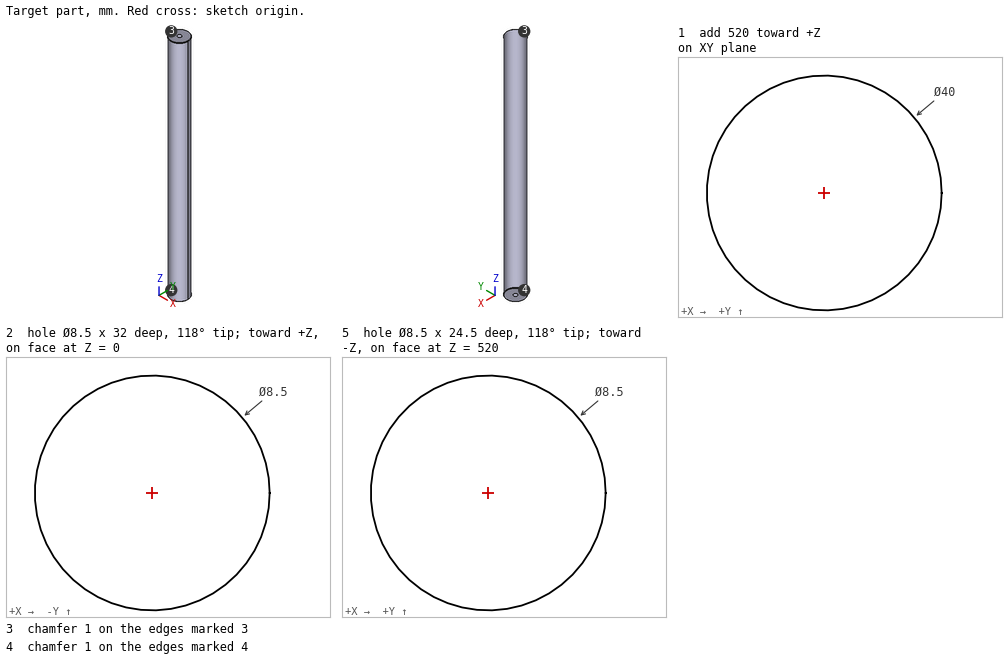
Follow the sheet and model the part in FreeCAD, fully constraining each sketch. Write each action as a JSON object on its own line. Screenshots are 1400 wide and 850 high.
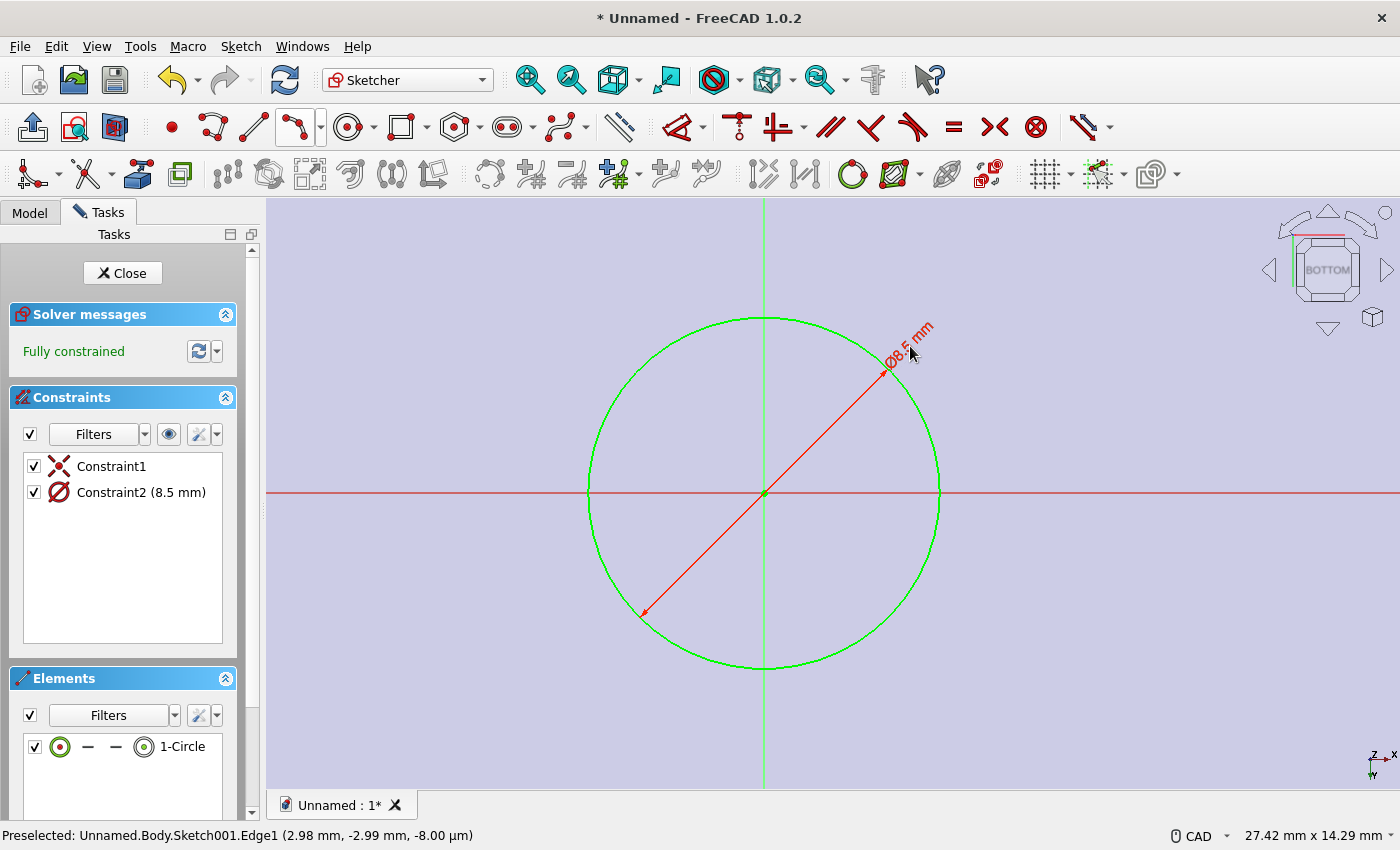
{"action": "left_click", "coordinate": [123, 273]}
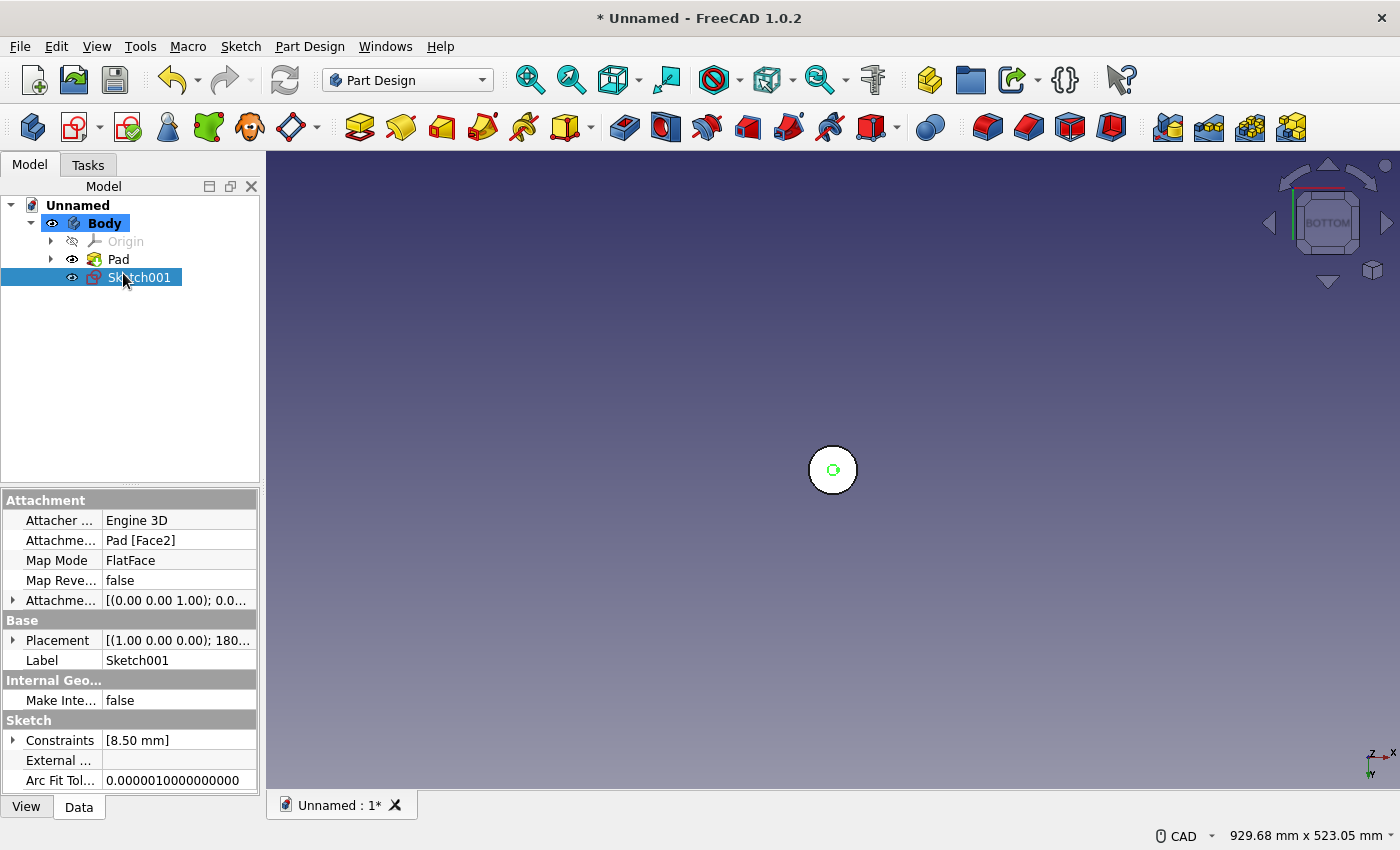
{"action": "left_click", "coordinate": [666, 128]}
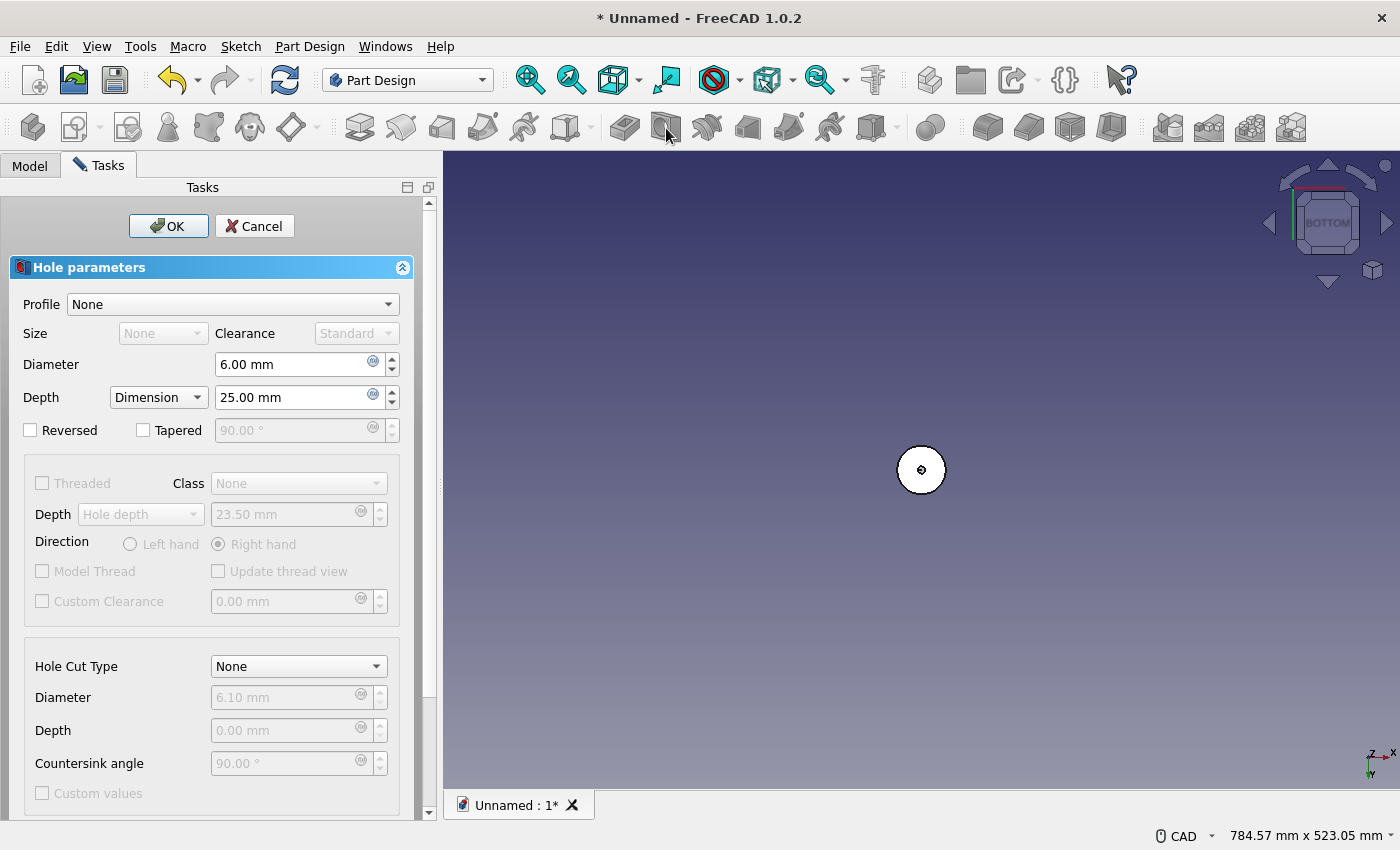
{"action": "triple_click", "coordinate": [300, 364]}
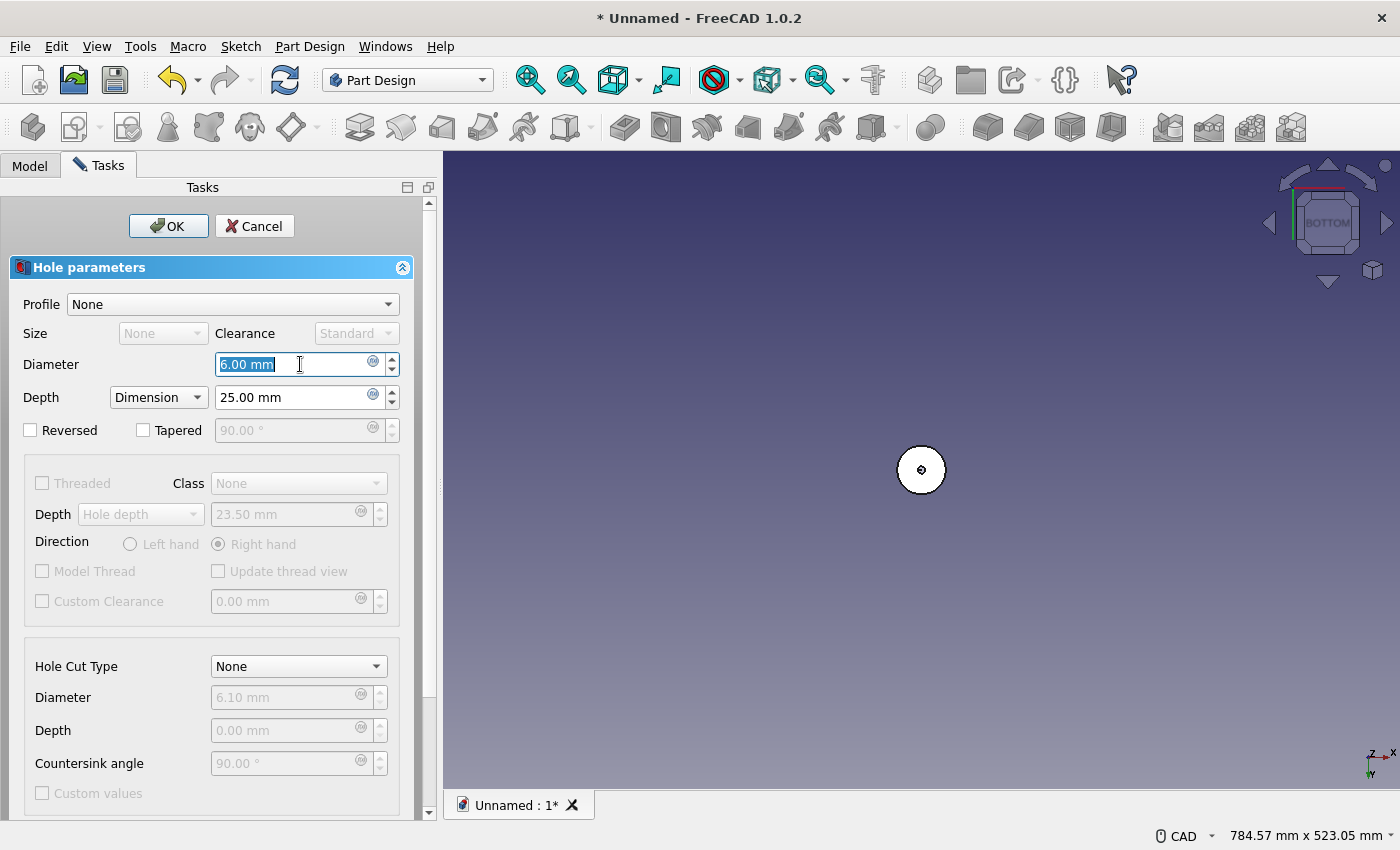
{"action": "type", "text": "8.5"}
{"action": "key", "text": "Tab"}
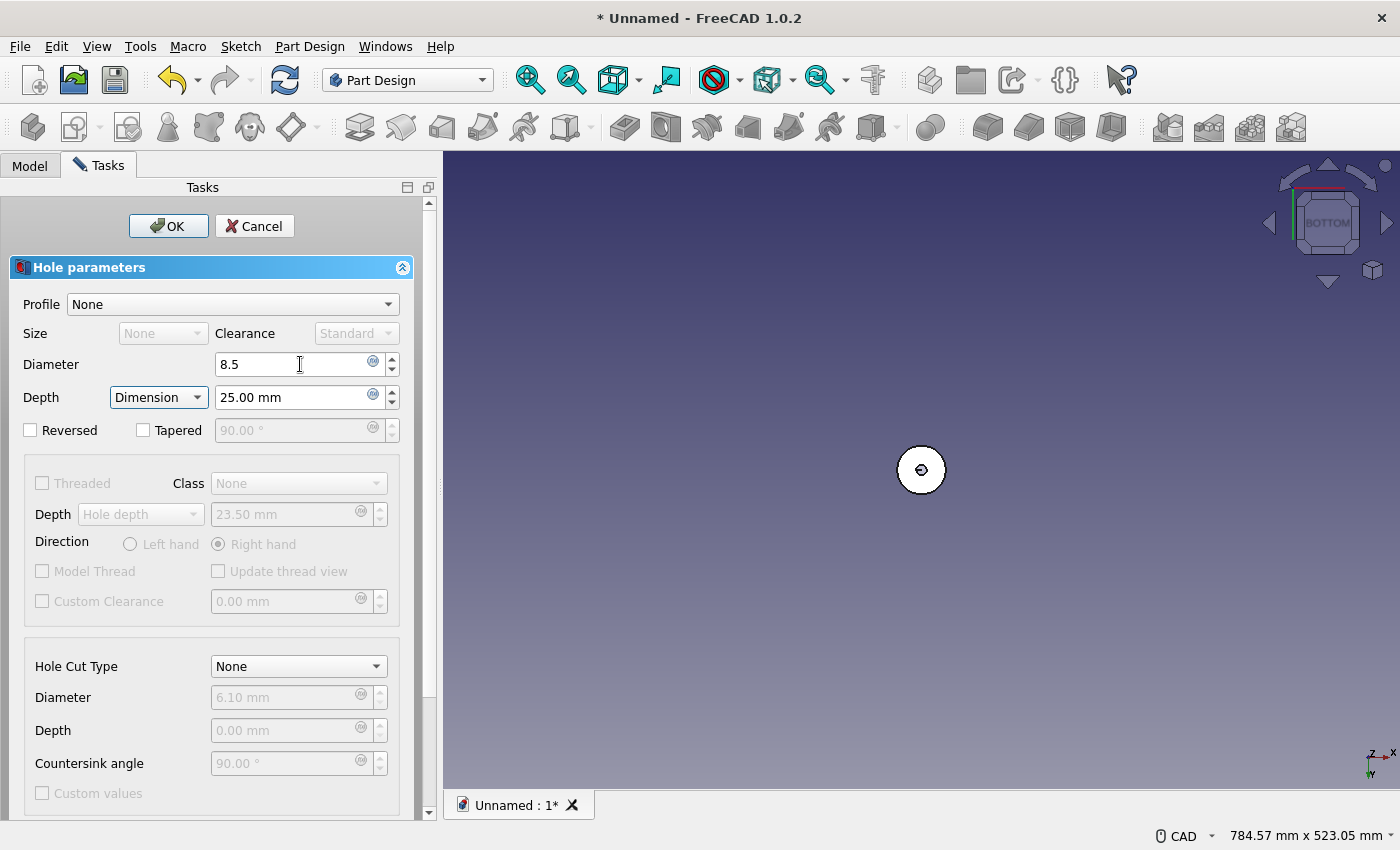
{"action": "triple_click", "coordinate": [300, 398]}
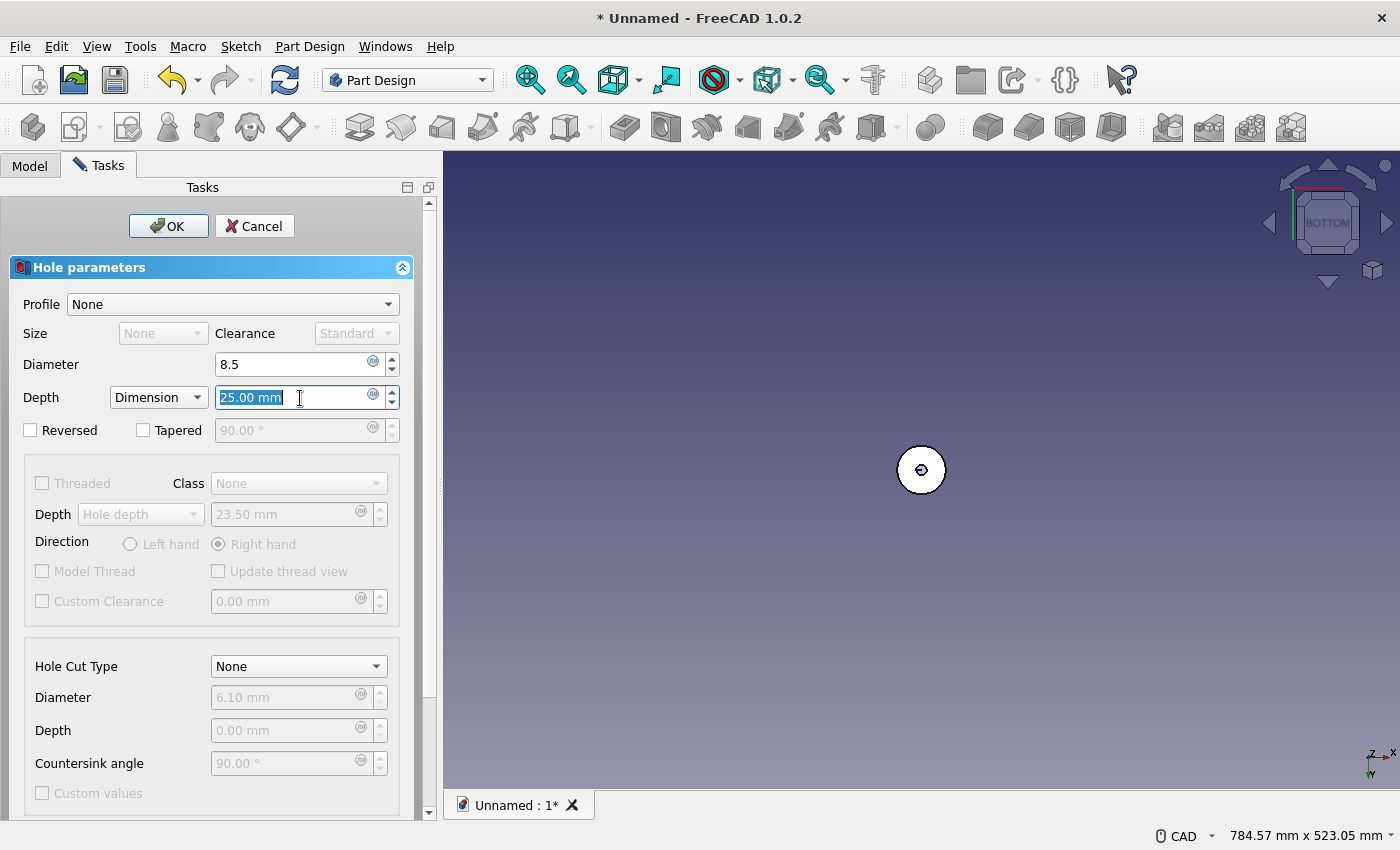
{"action": "type", "text": "32"}
{"action": "key", "text": "Tab"}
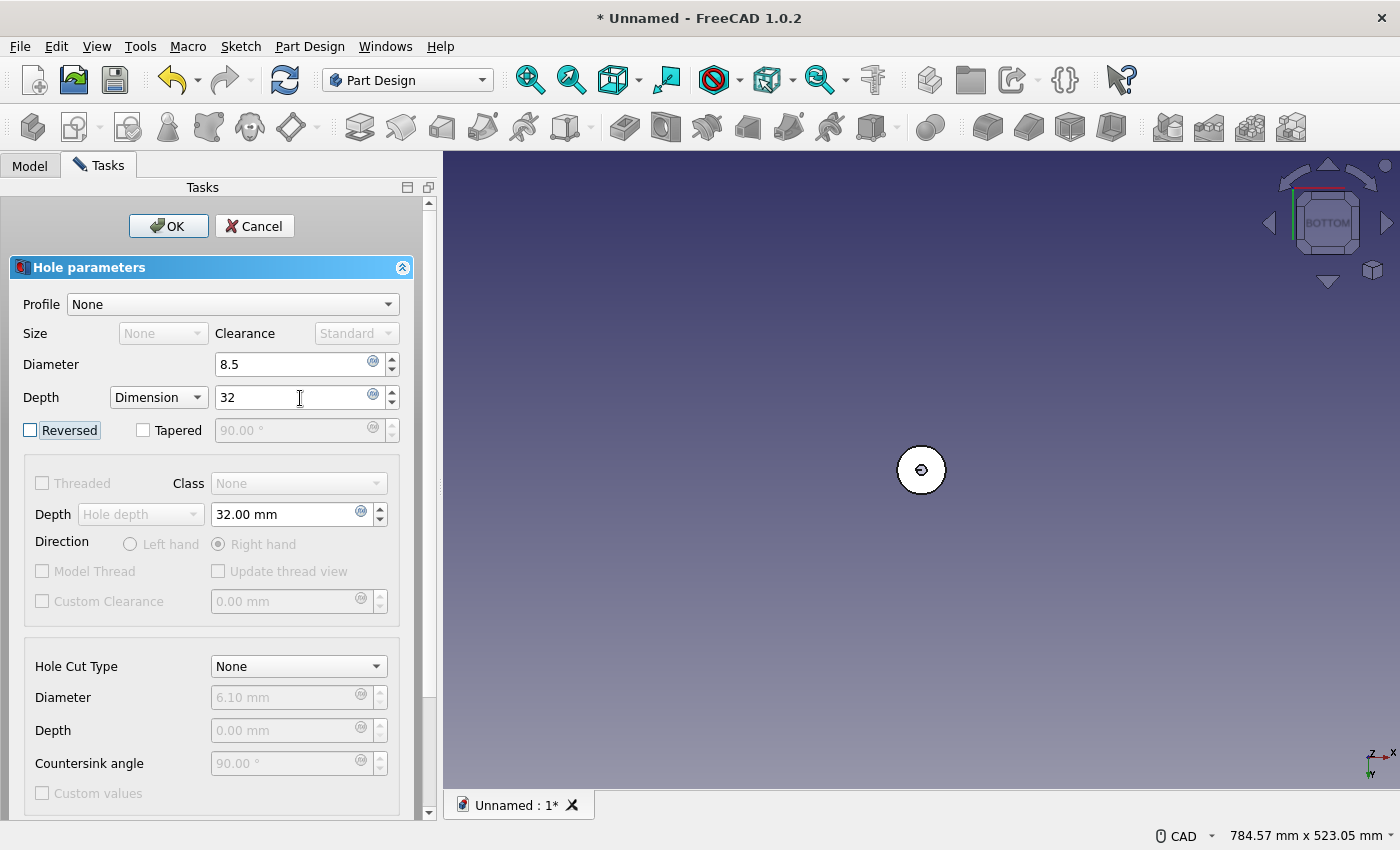
{"action": "left_click", "coordinate": [169, 226]}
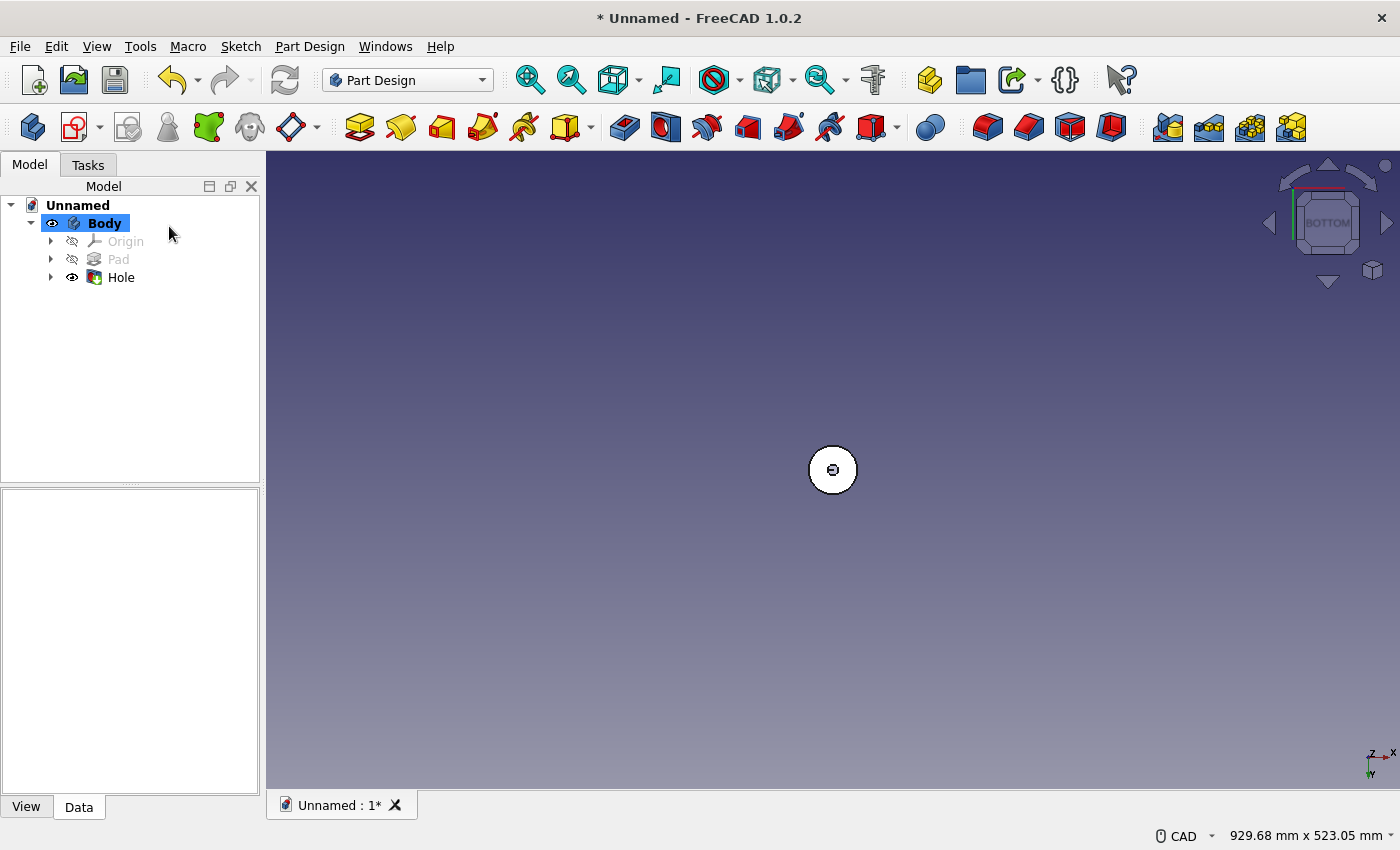
{"action": "left_click", "coordinate": [531, 80]}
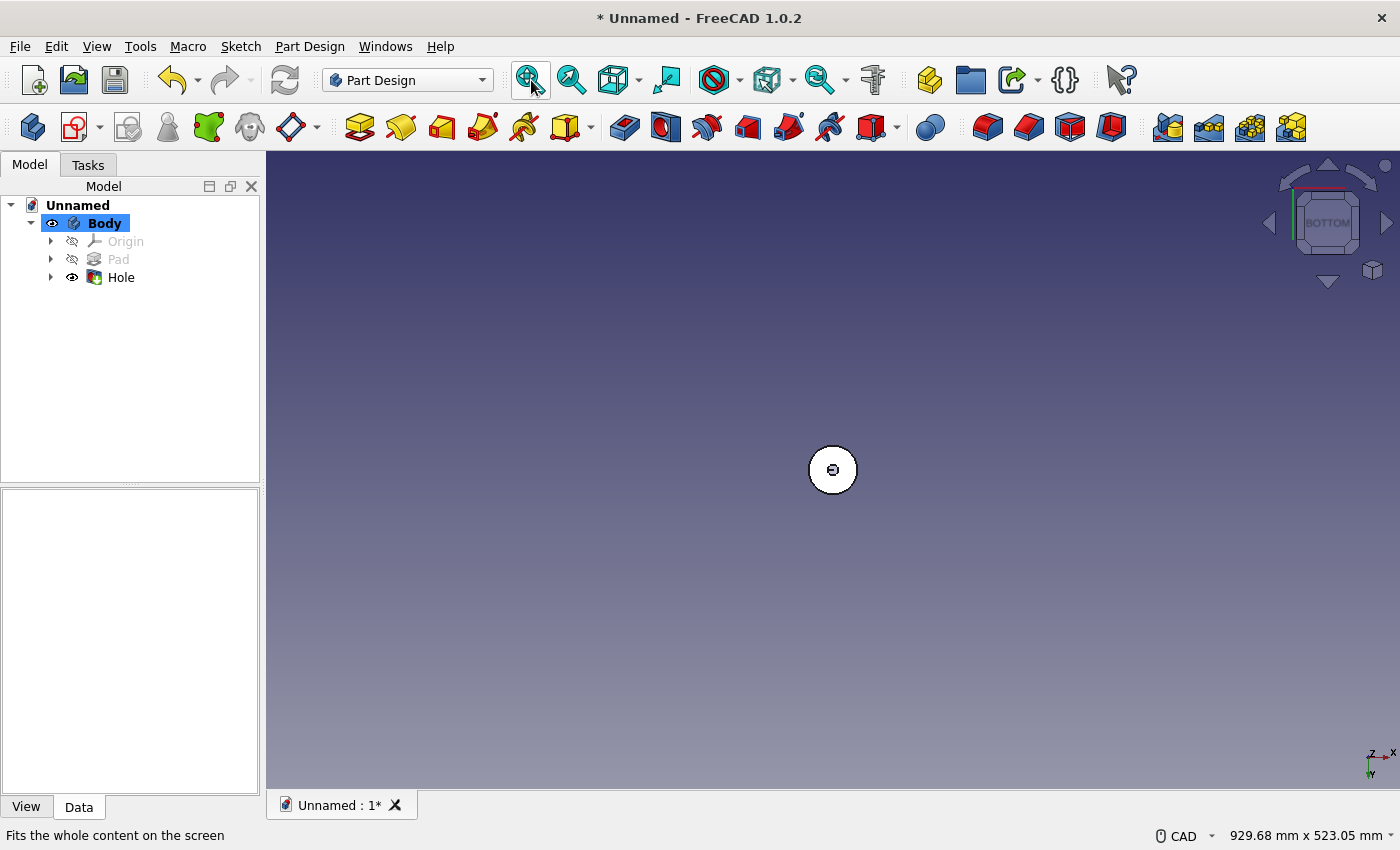
{"action": "key", "text": "0"}